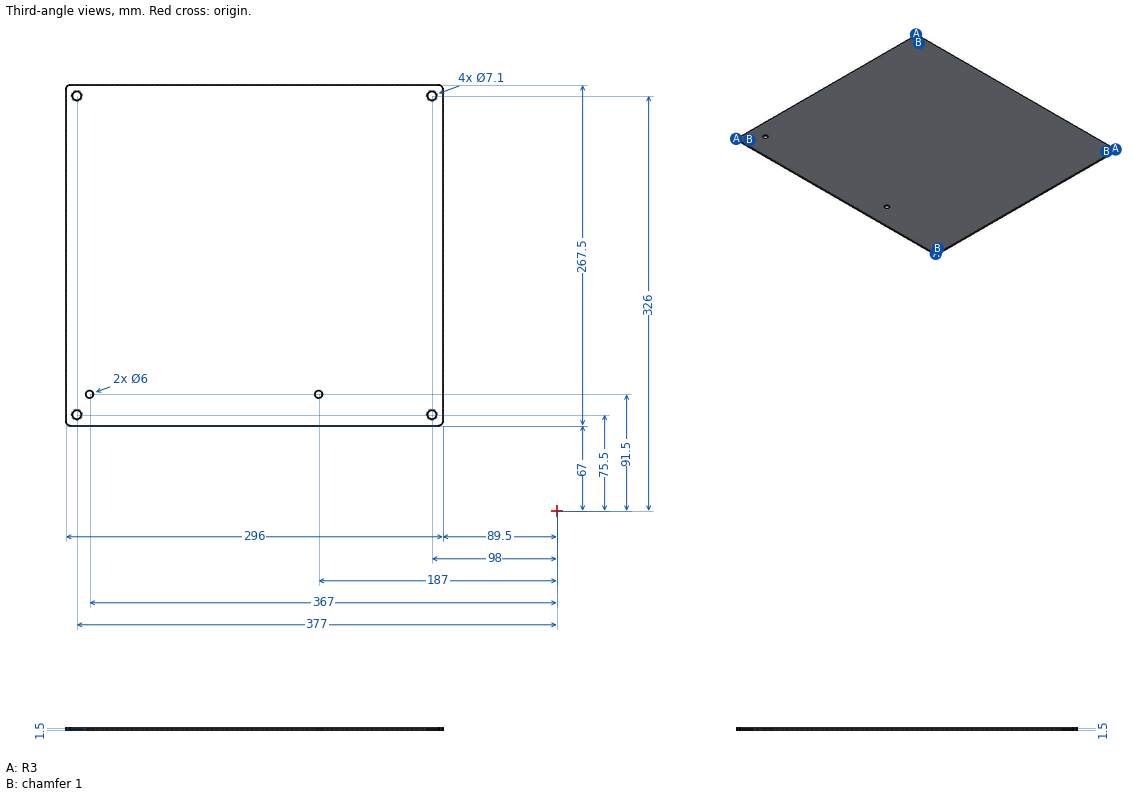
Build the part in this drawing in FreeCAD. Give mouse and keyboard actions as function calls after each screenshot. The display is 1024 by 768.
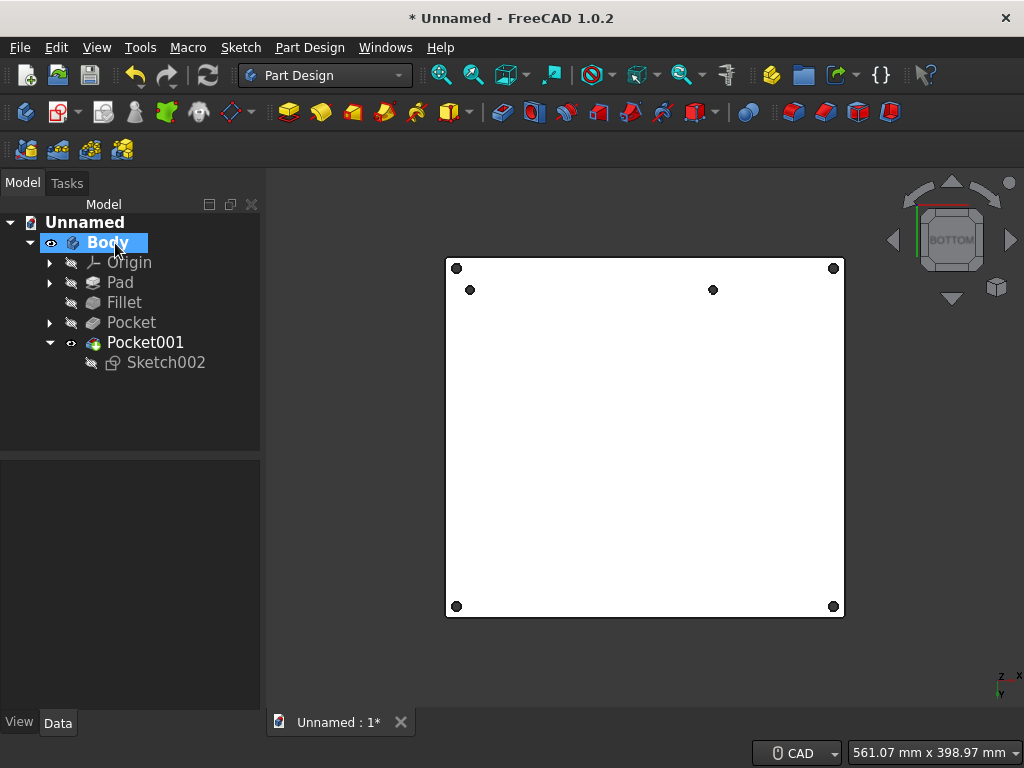
click(829, 606)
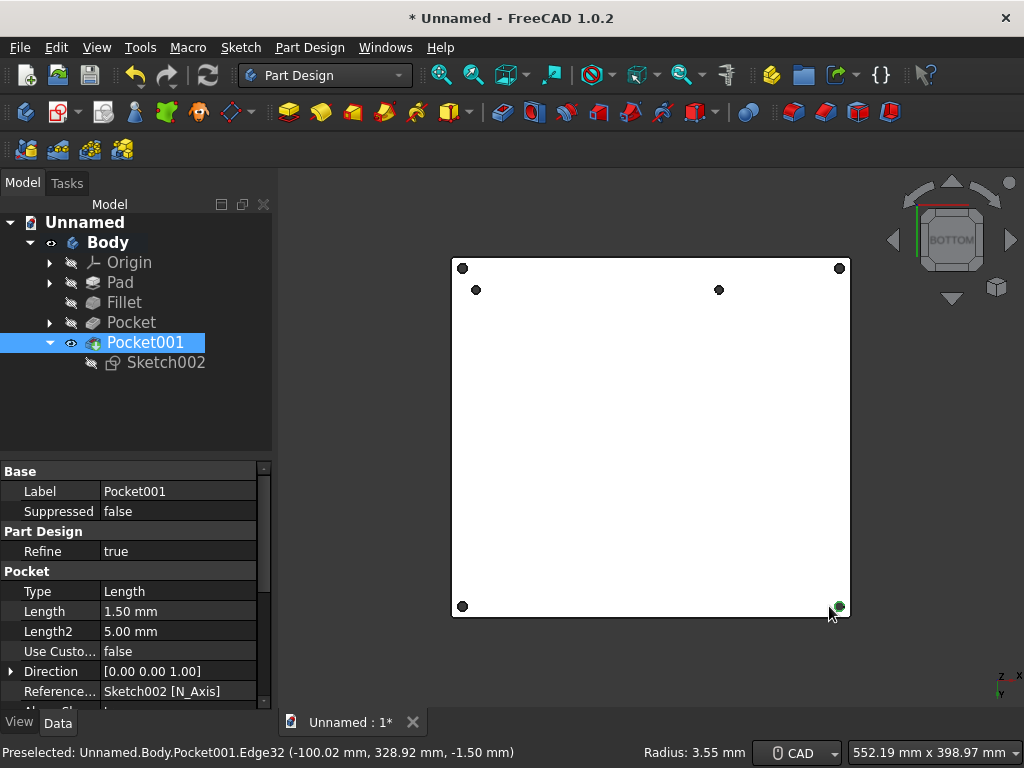
click(458, 606, ctrl)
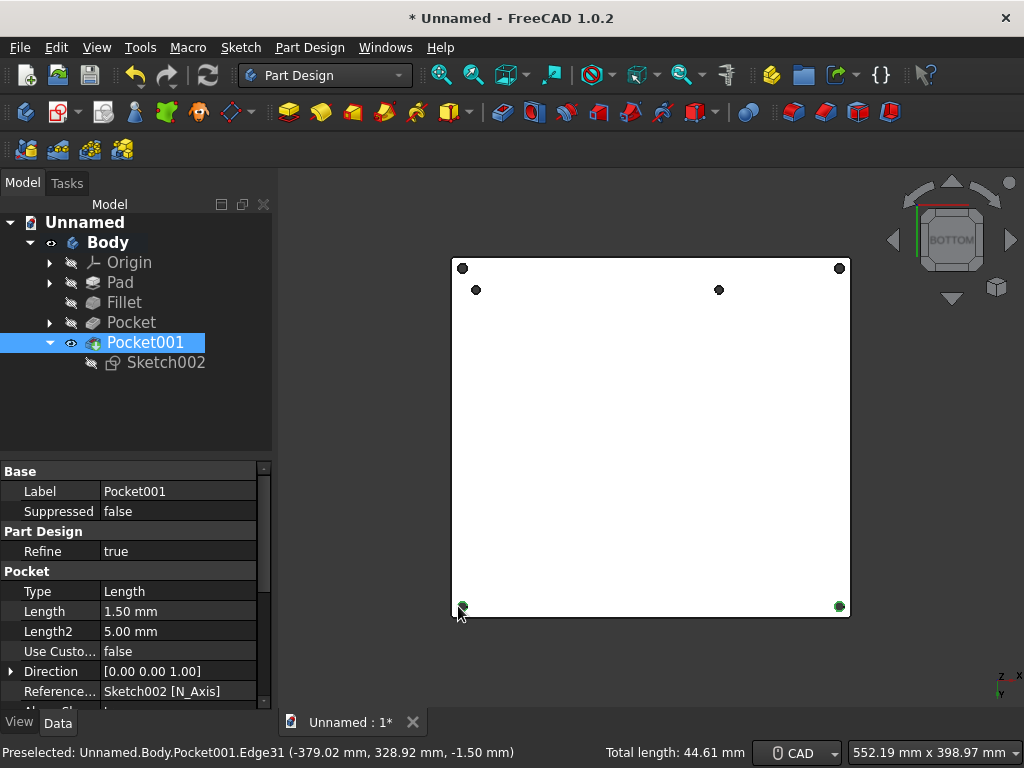
click(458, 267, ctrl)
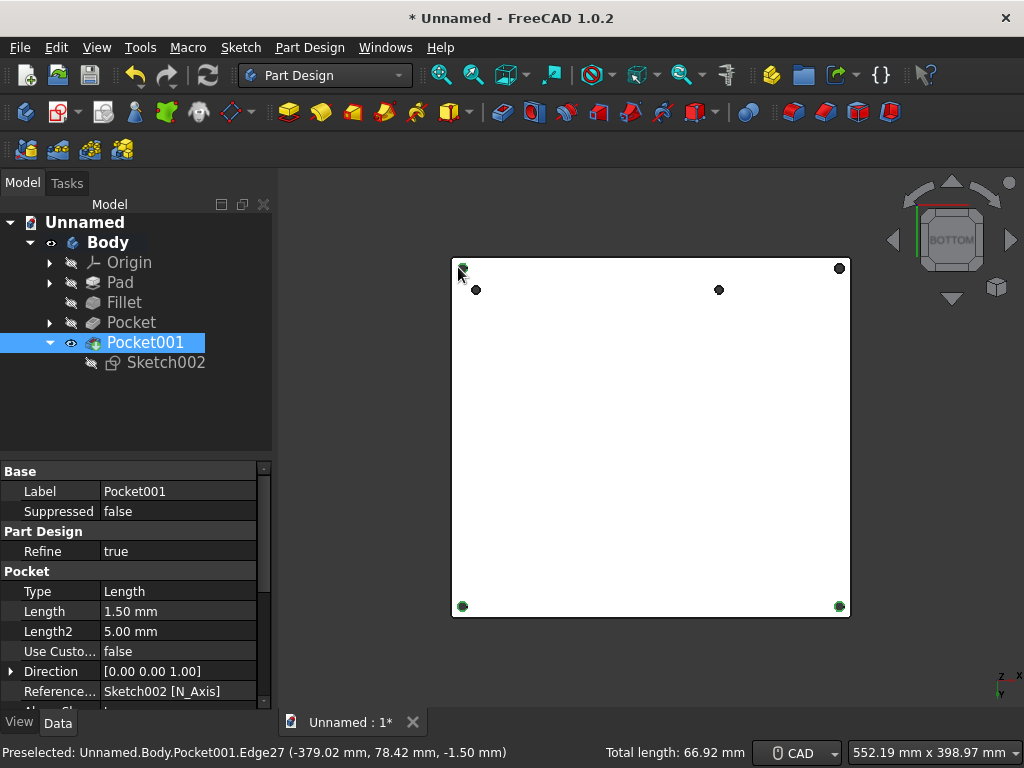
click(835, 267, ctrl)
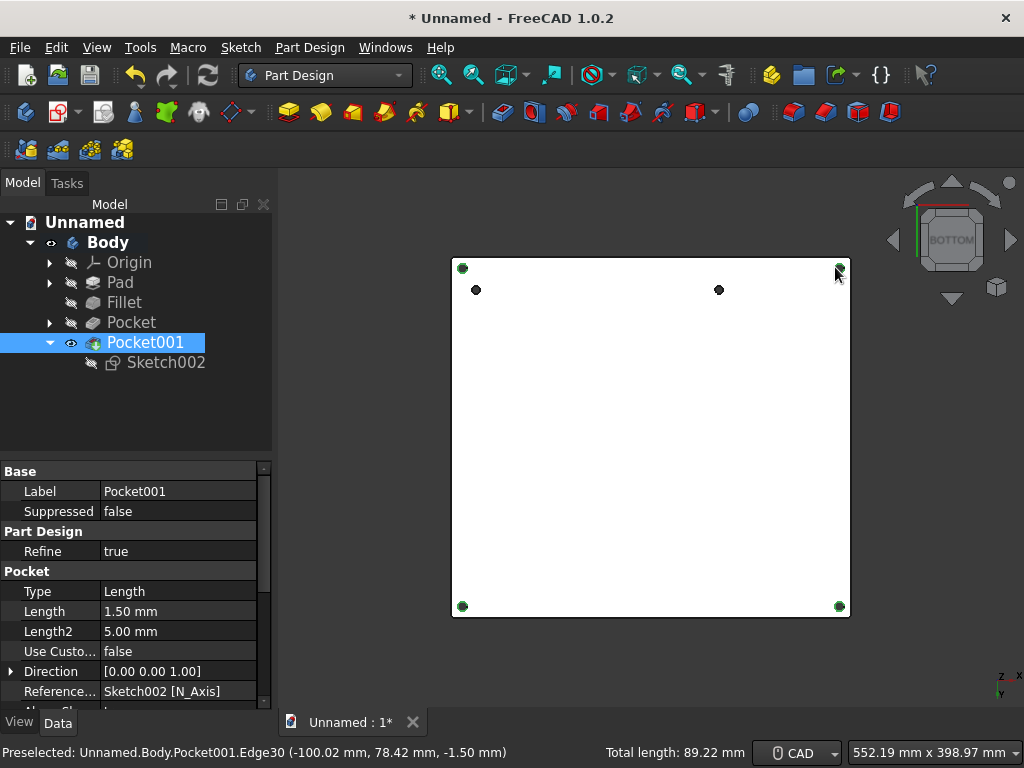
click(826, 112)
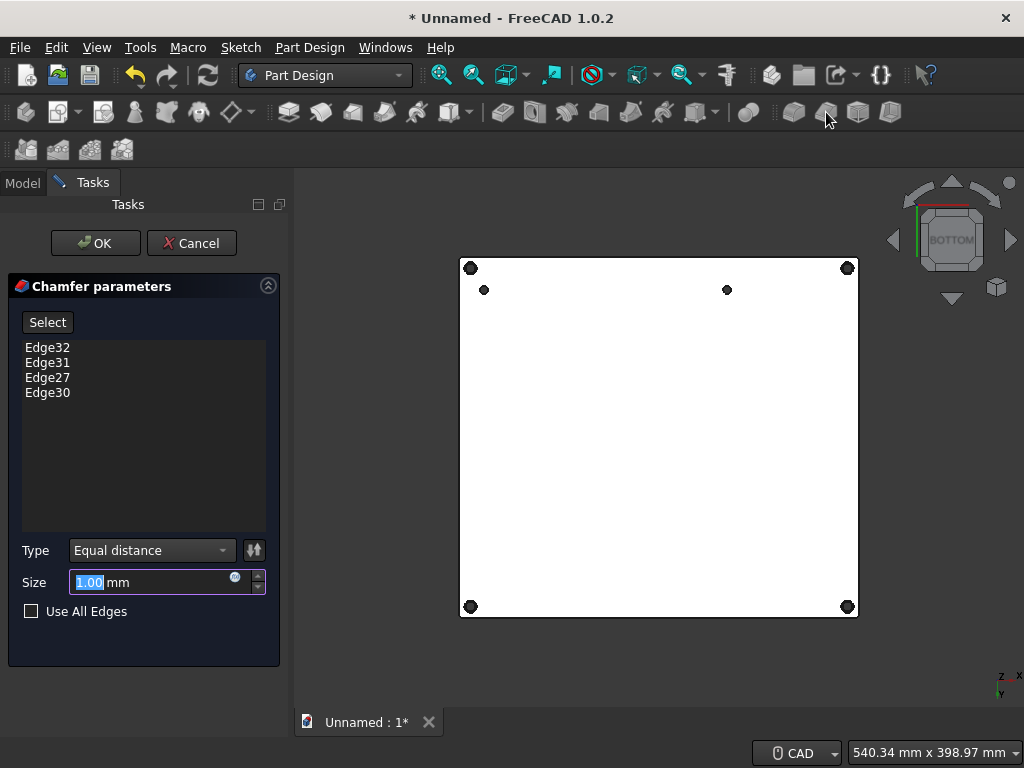
text(1)
key(Tab)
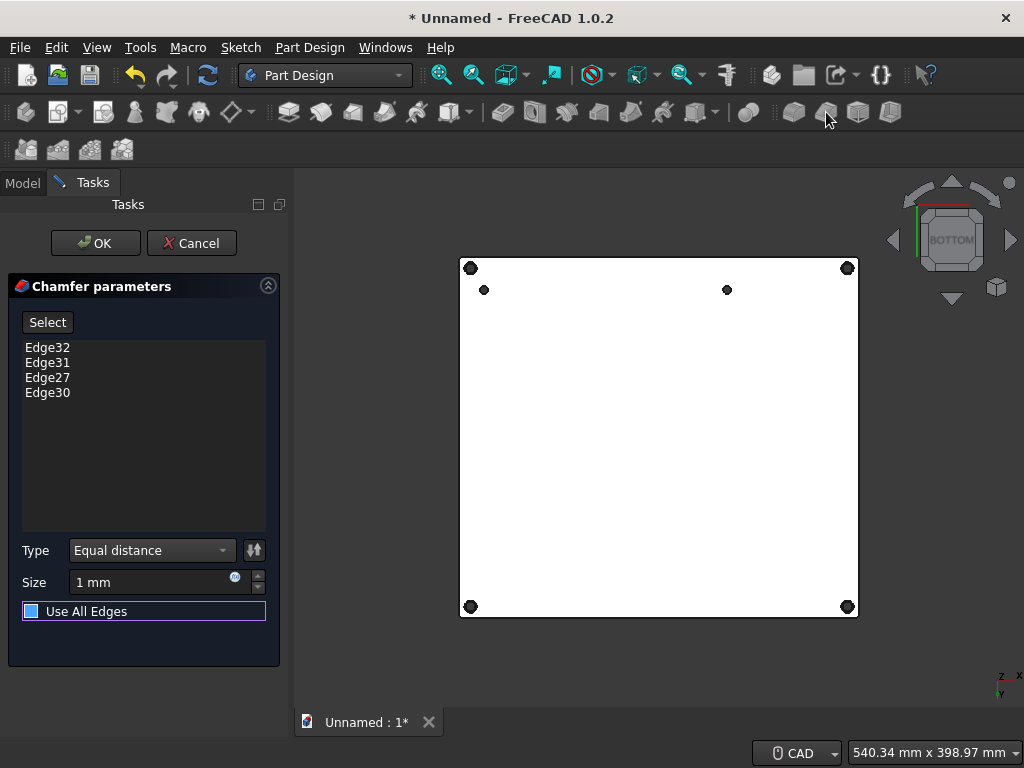
click(96, 243)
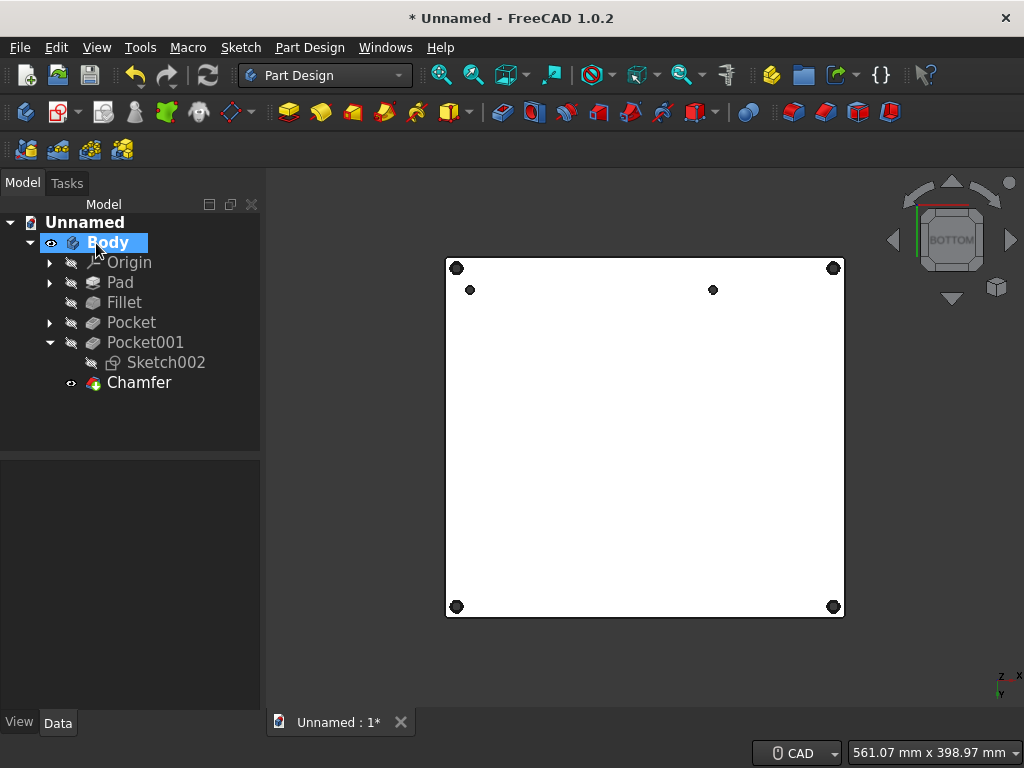
key(0)